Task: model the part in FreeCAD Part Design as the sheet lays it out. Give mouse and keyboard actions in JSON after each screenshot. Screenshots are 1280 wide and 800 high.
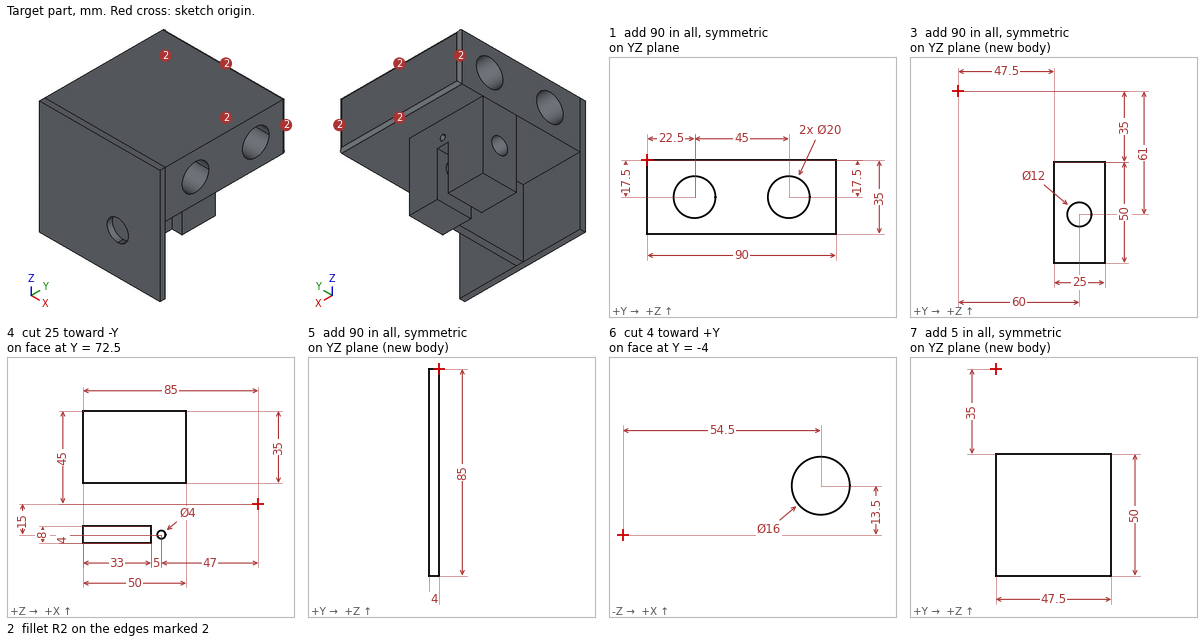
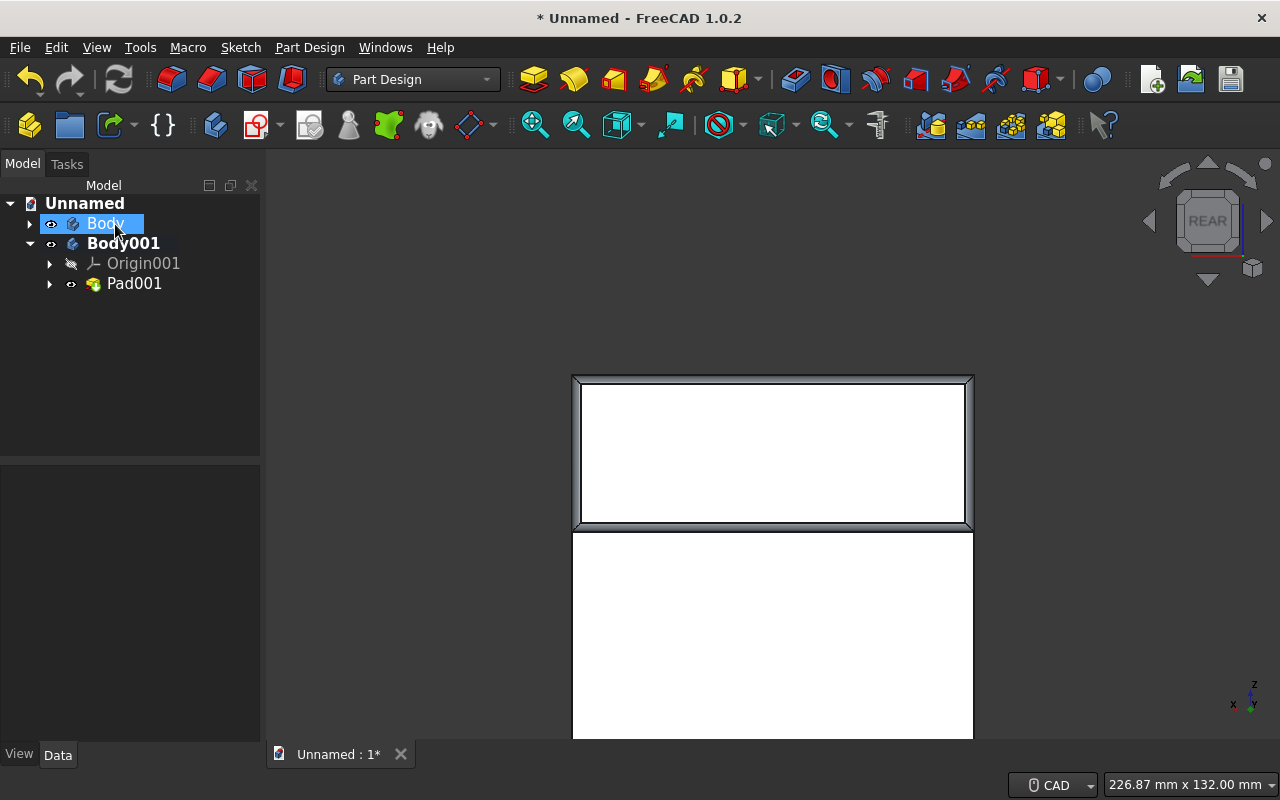
{"action": "key", "text": "v f"}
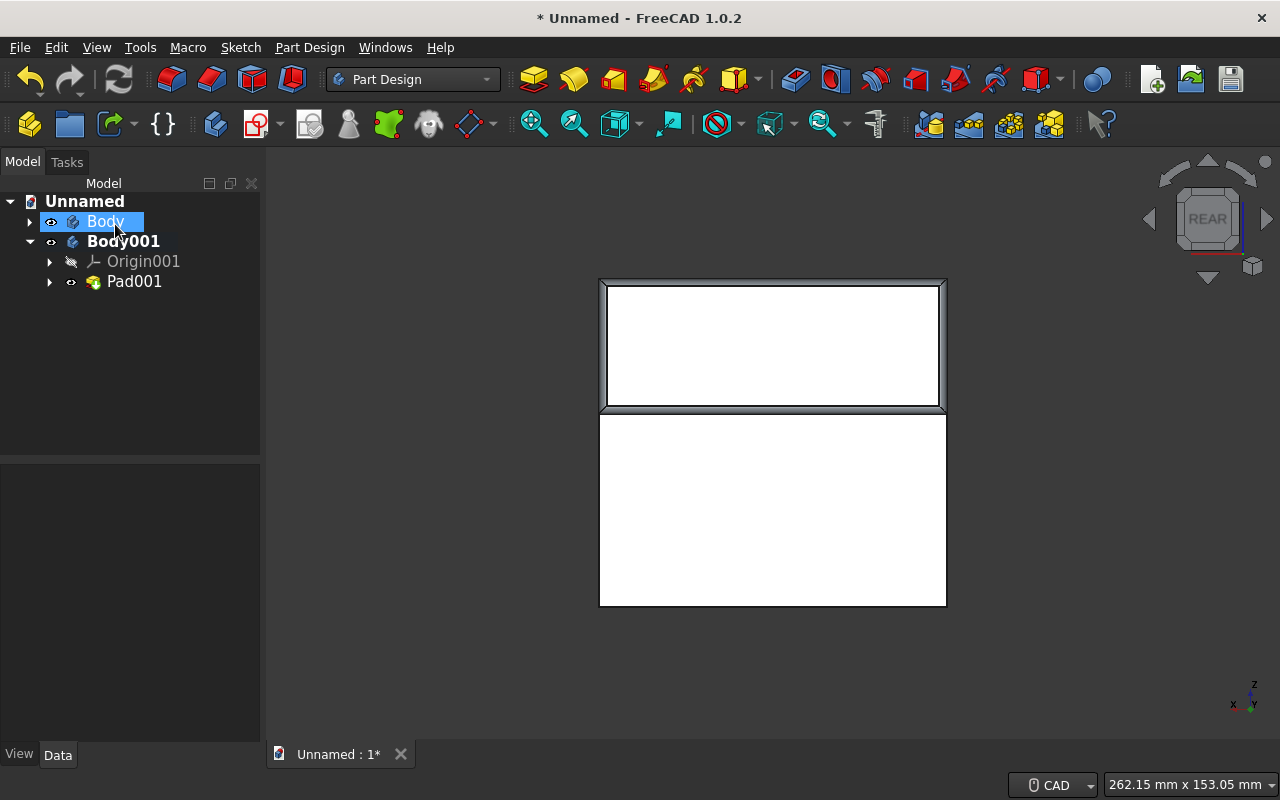
{"action": "left_click", "coordinate": [823, 510]}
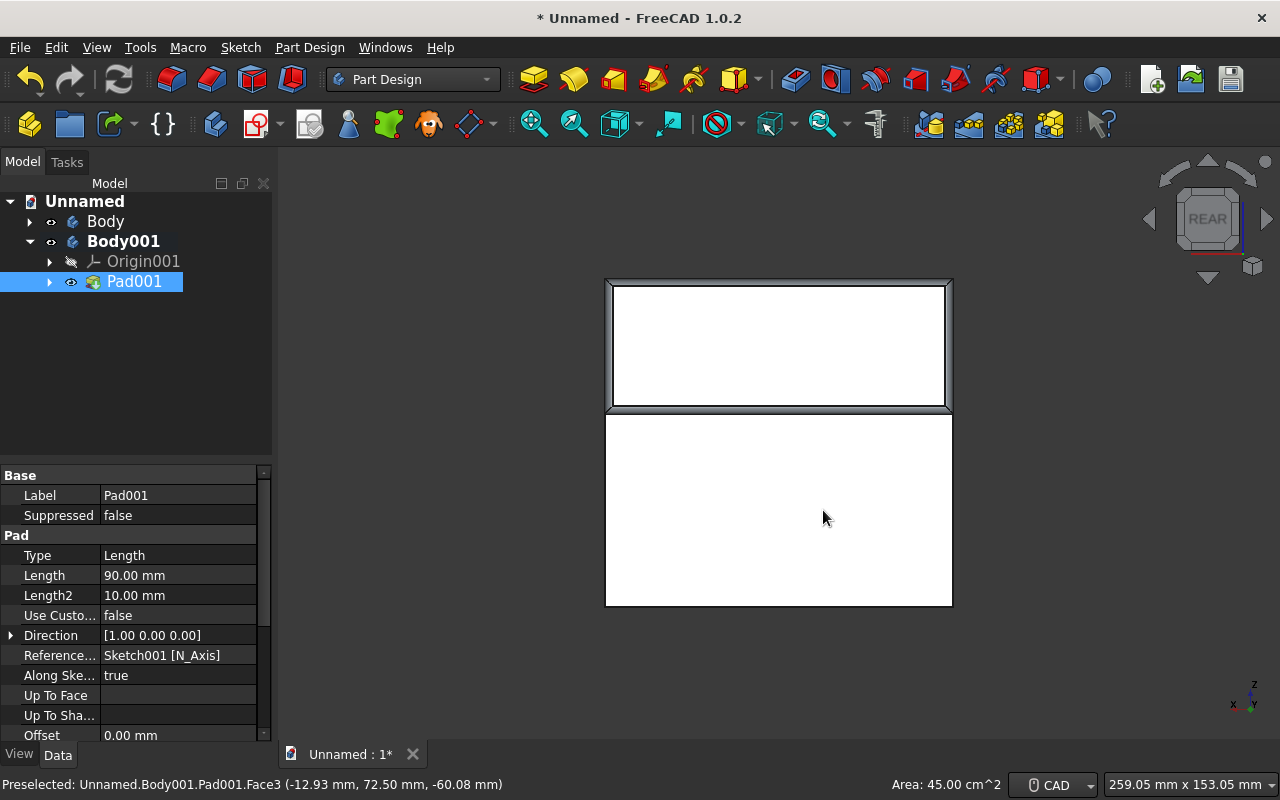
{"action": "left_click", "coordinate": [256, 124]}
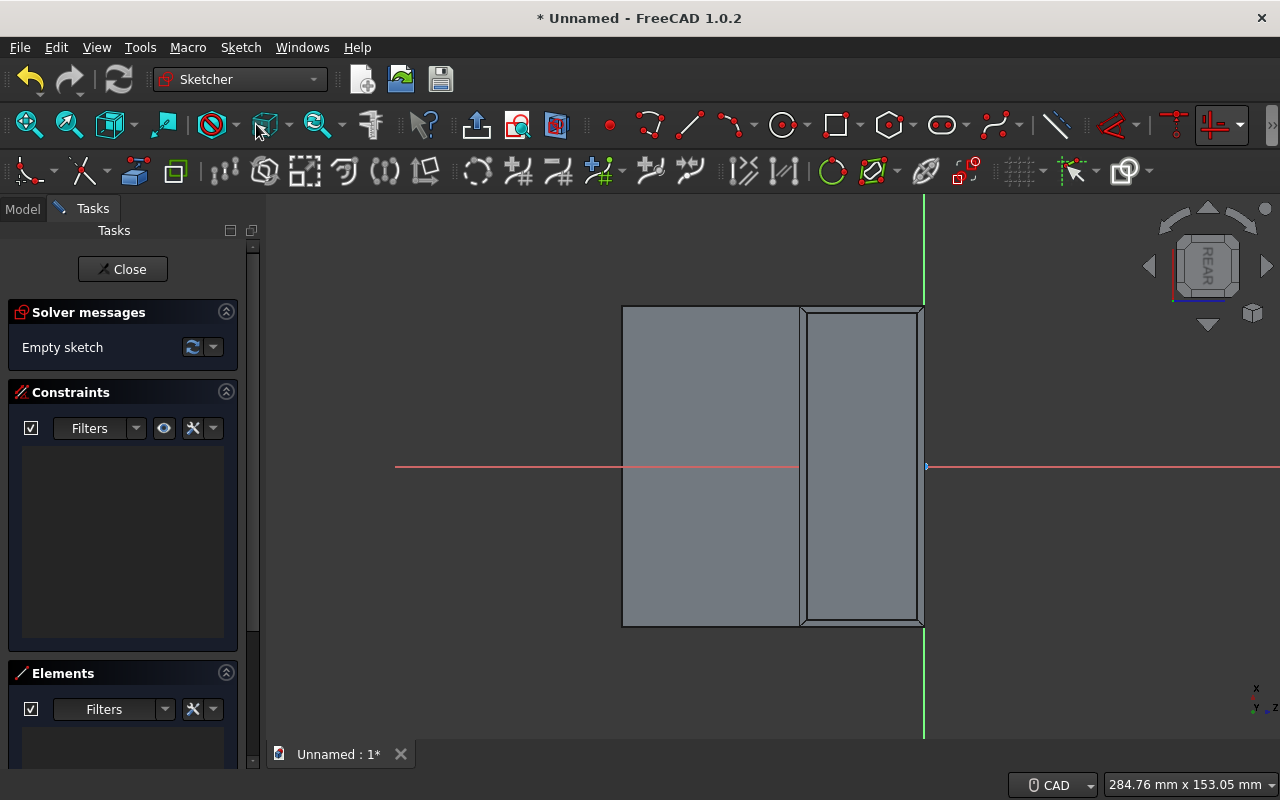
{"action": "scroll", "coordinate": [912, 326], "scroll_direction": "up", "scroll_amount": 2}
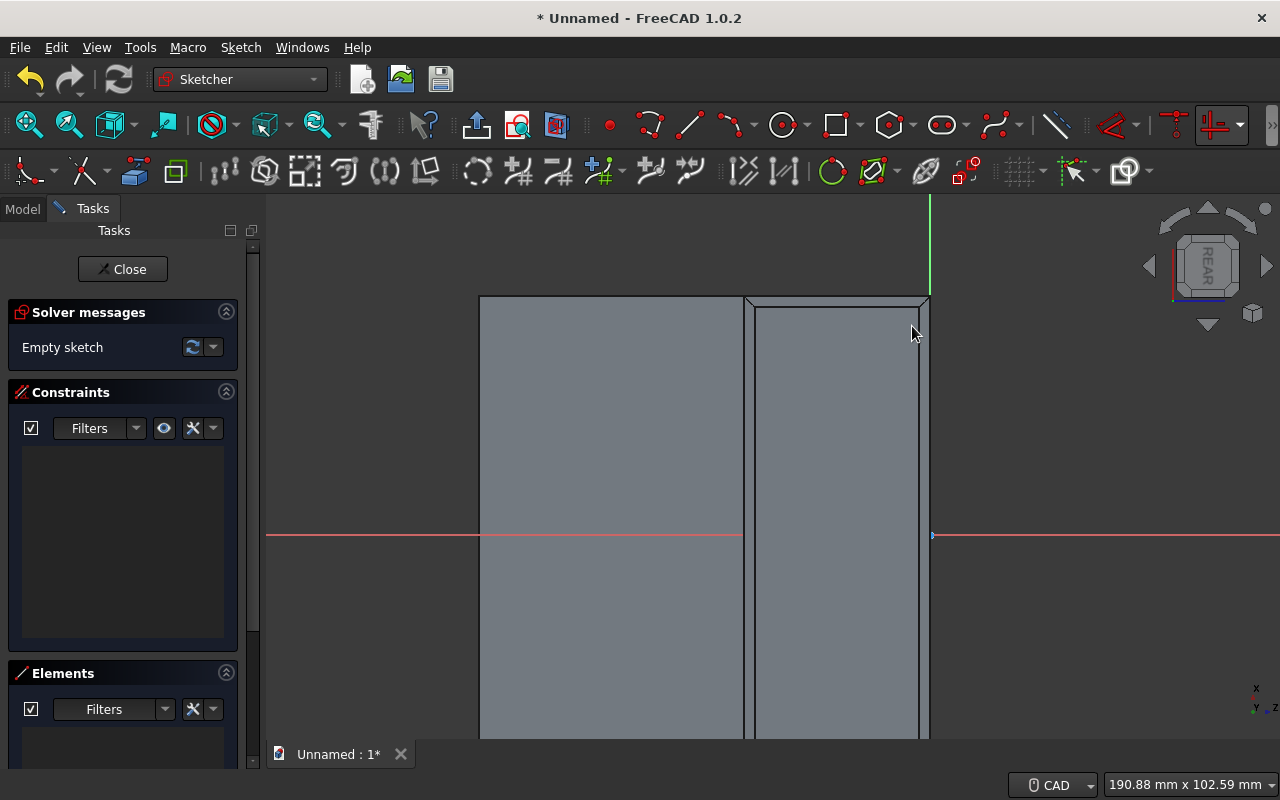
{"action": "left_click", "coordinate": [836, 126]}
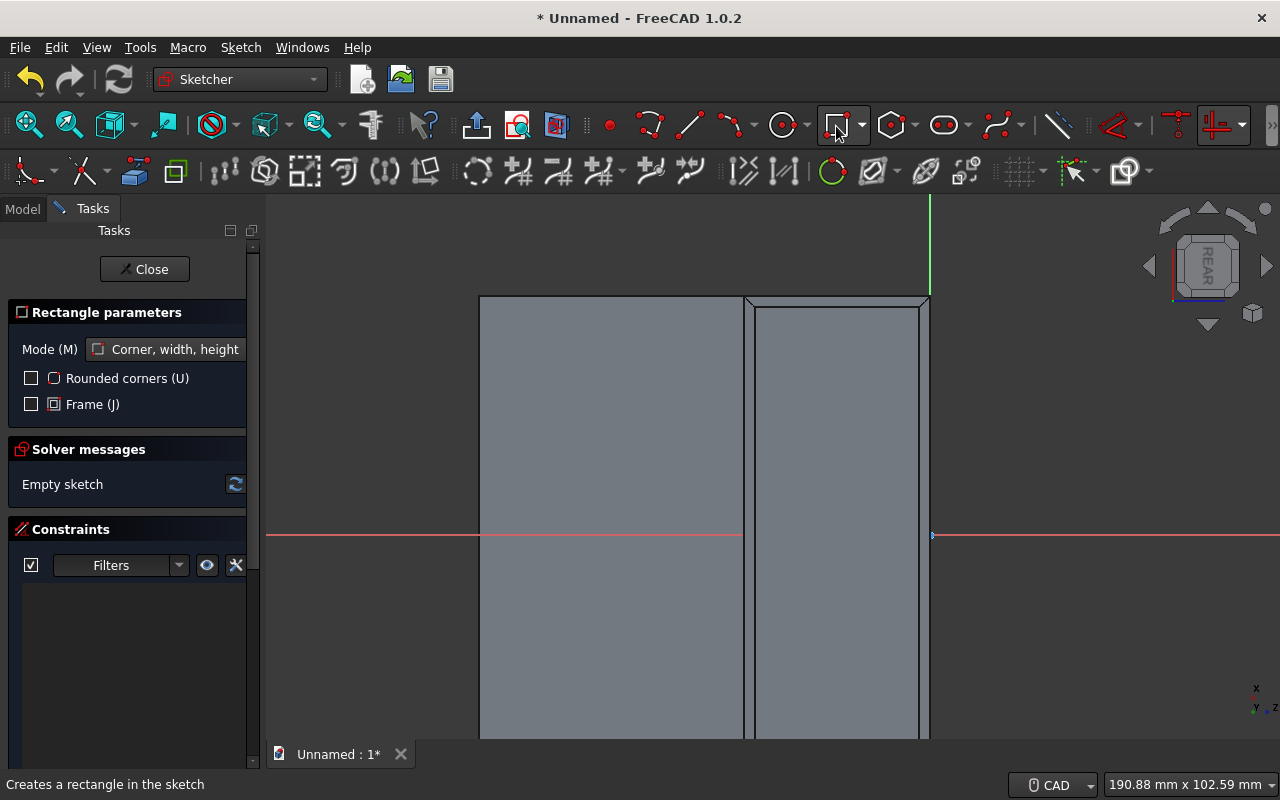
{"action": "left_click", "coordinate": [479, 296]}
{"action": "mouse_move", "coordinate": [744, 482]}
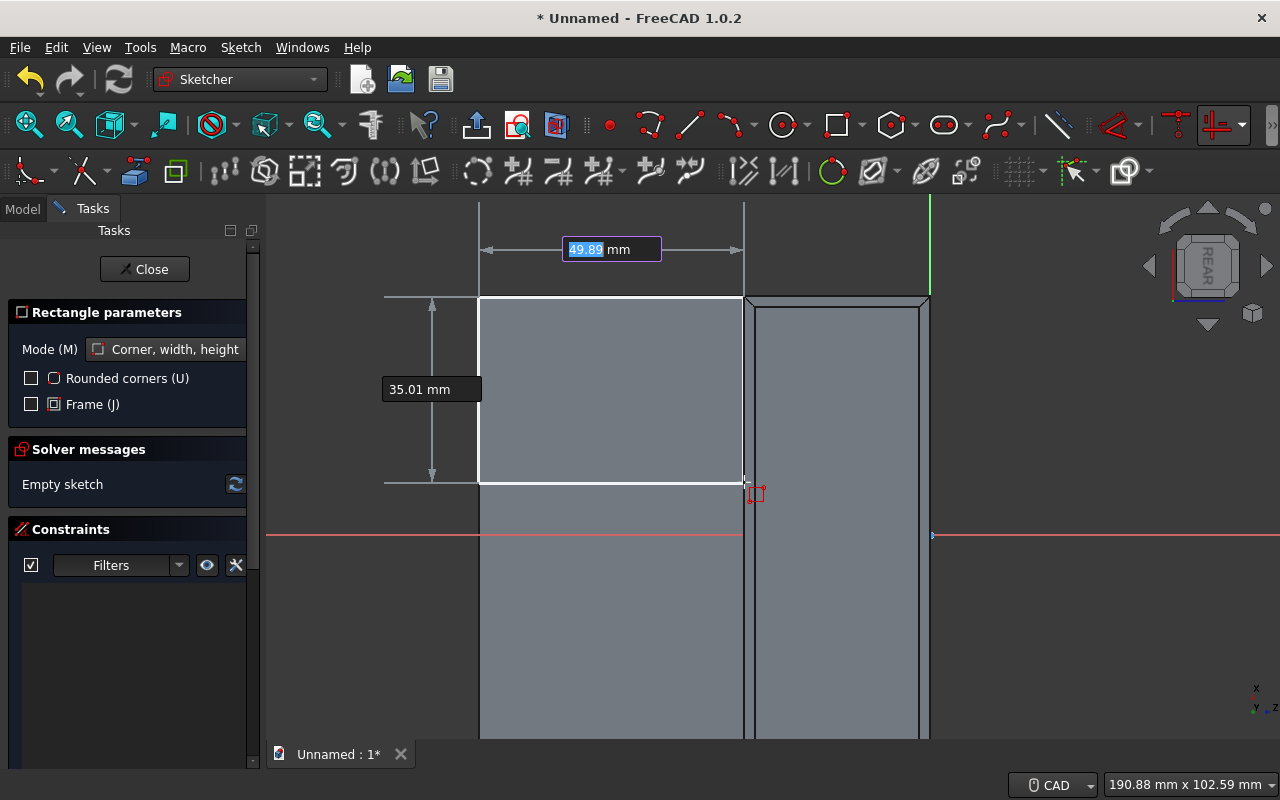
{"action": "type", "text": "50"}
{"action": "key", "text": "Tab"}
{"action": "type", "text": "35"}
{"action": "key", "text": "Return"}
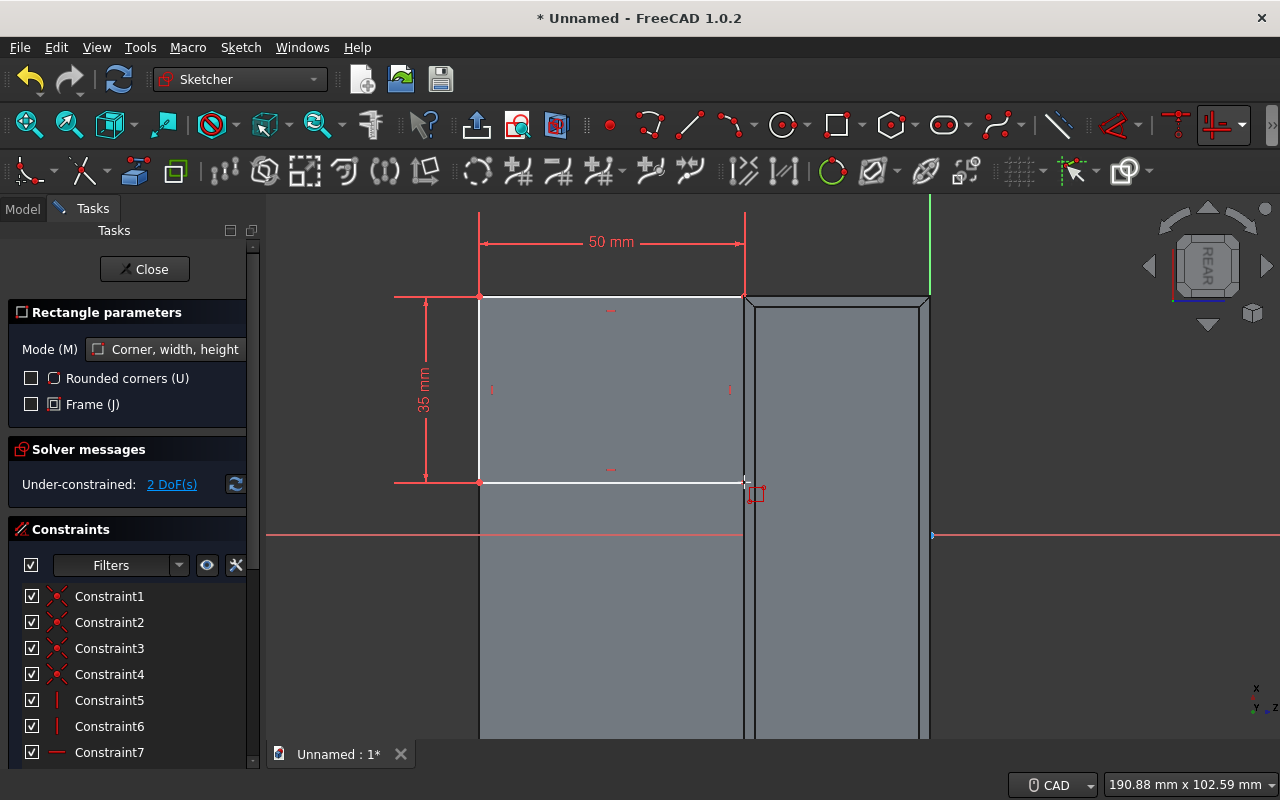
{"action": "left_click", "coordinate": [479, 594]}
{"action": "mouse_move", "coordinate": [654, 636]}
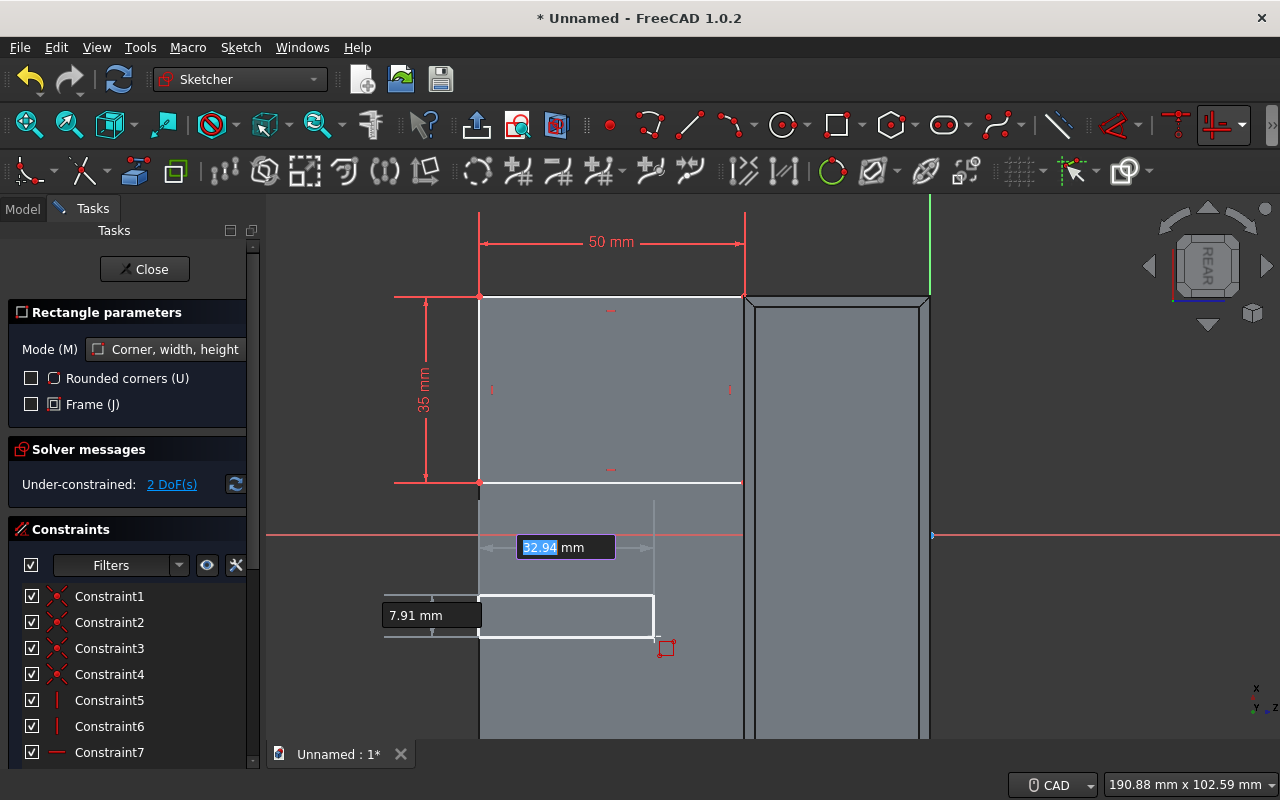
{"action": "type", "text": "33"}
{"action": "key", "text": "Tab"}
{"action": "type", "text": "8"}
{"action": "key", "text": "Return"}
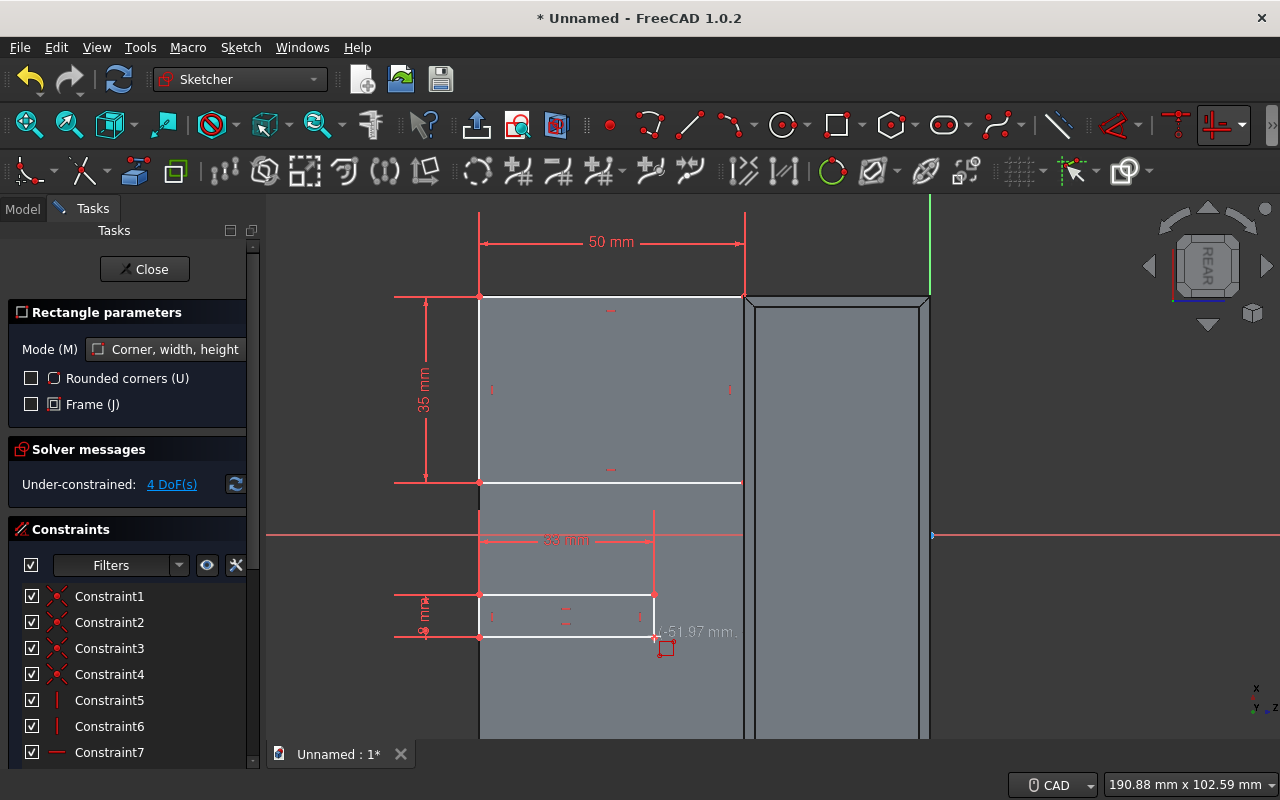
{"action": "left_click", "coordinate": [784, 126]}